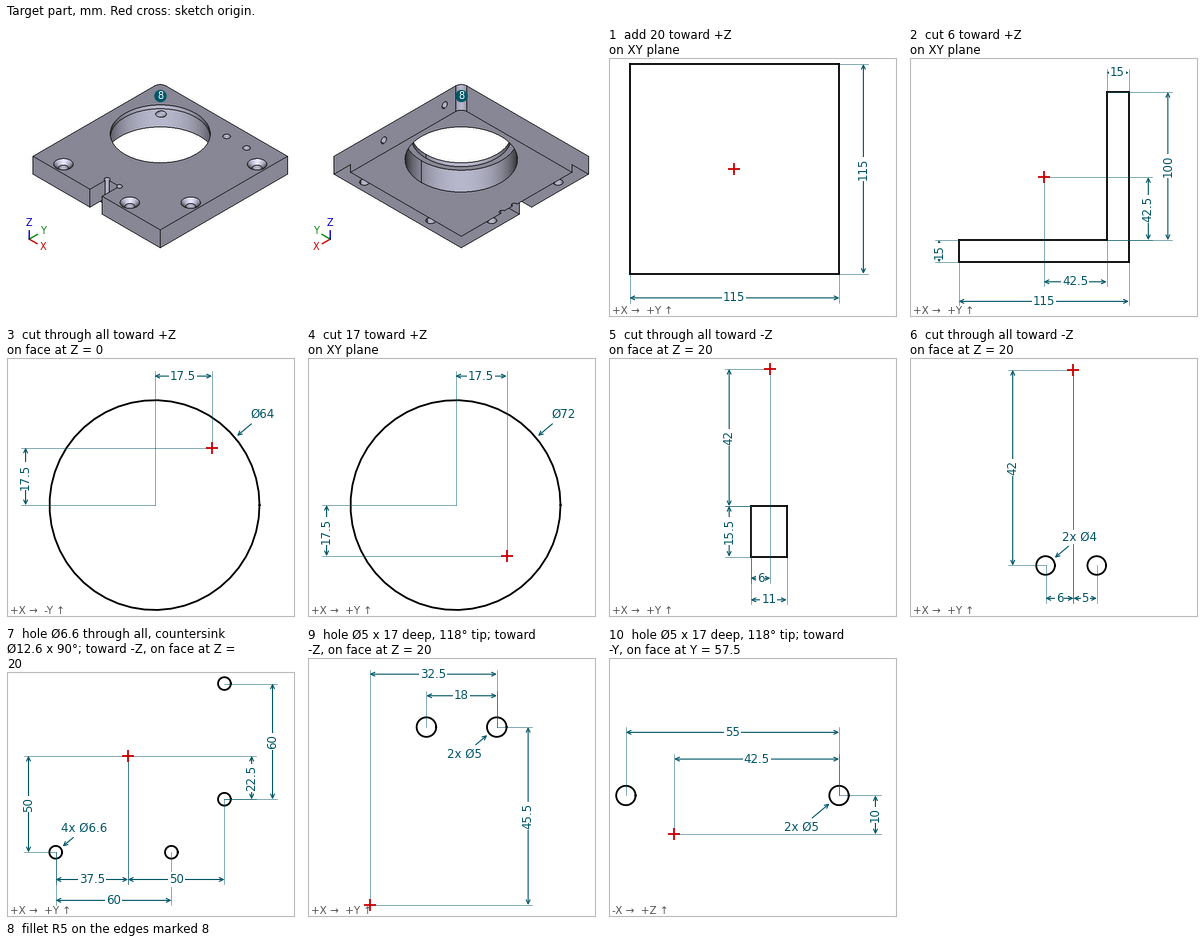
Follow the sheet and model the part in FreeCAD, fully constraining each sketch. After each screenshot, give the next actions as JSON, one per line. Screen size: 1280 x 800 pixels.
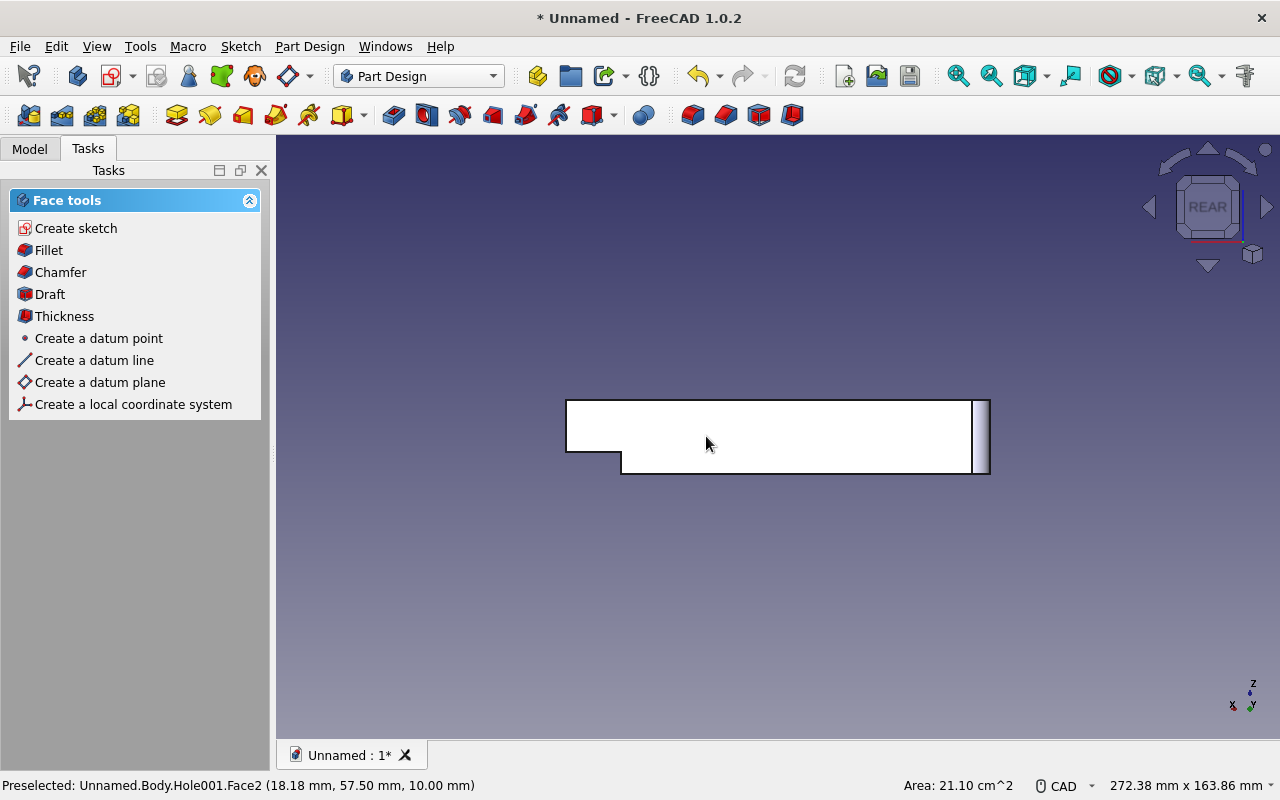
{"action": "left_click", "coordinate": [110, 76]}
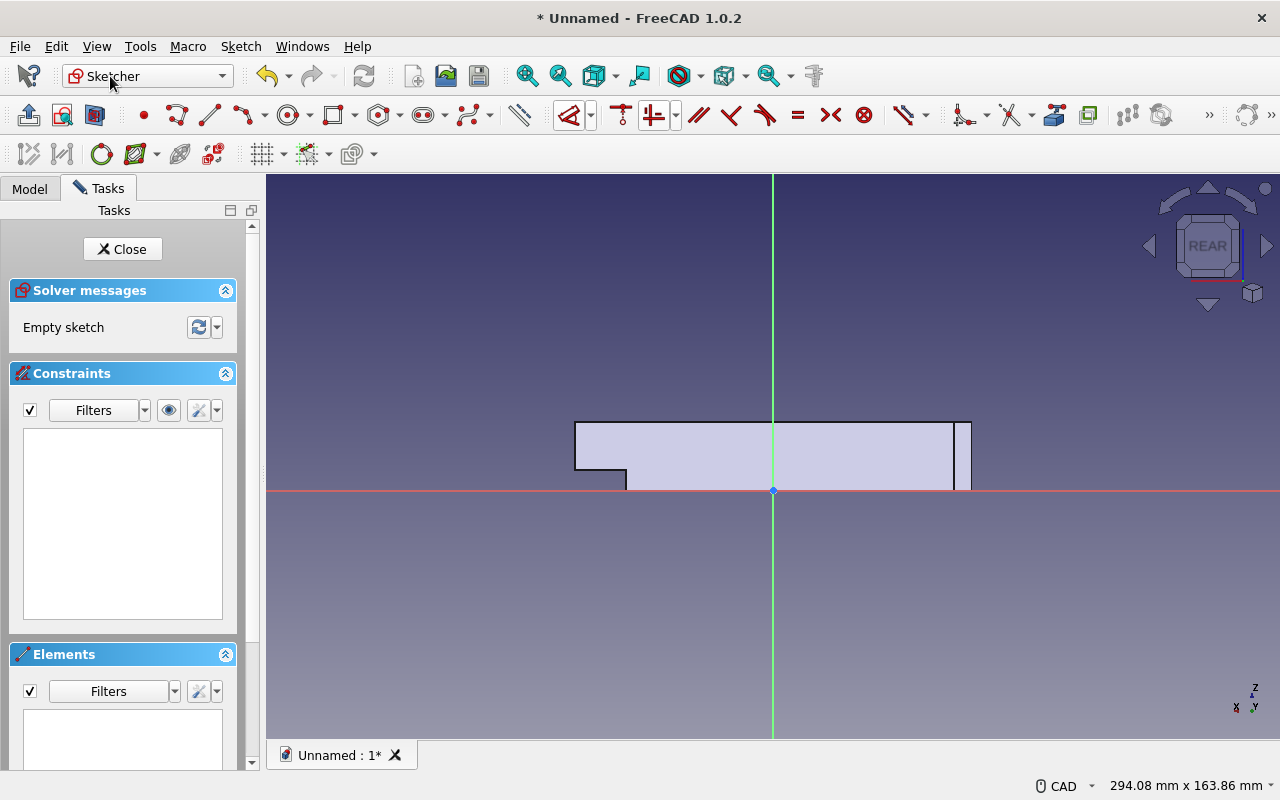
{"action": "scroll", "coordinate": [895, 477], "scroll_direction": "up", "scroll_amount": 5}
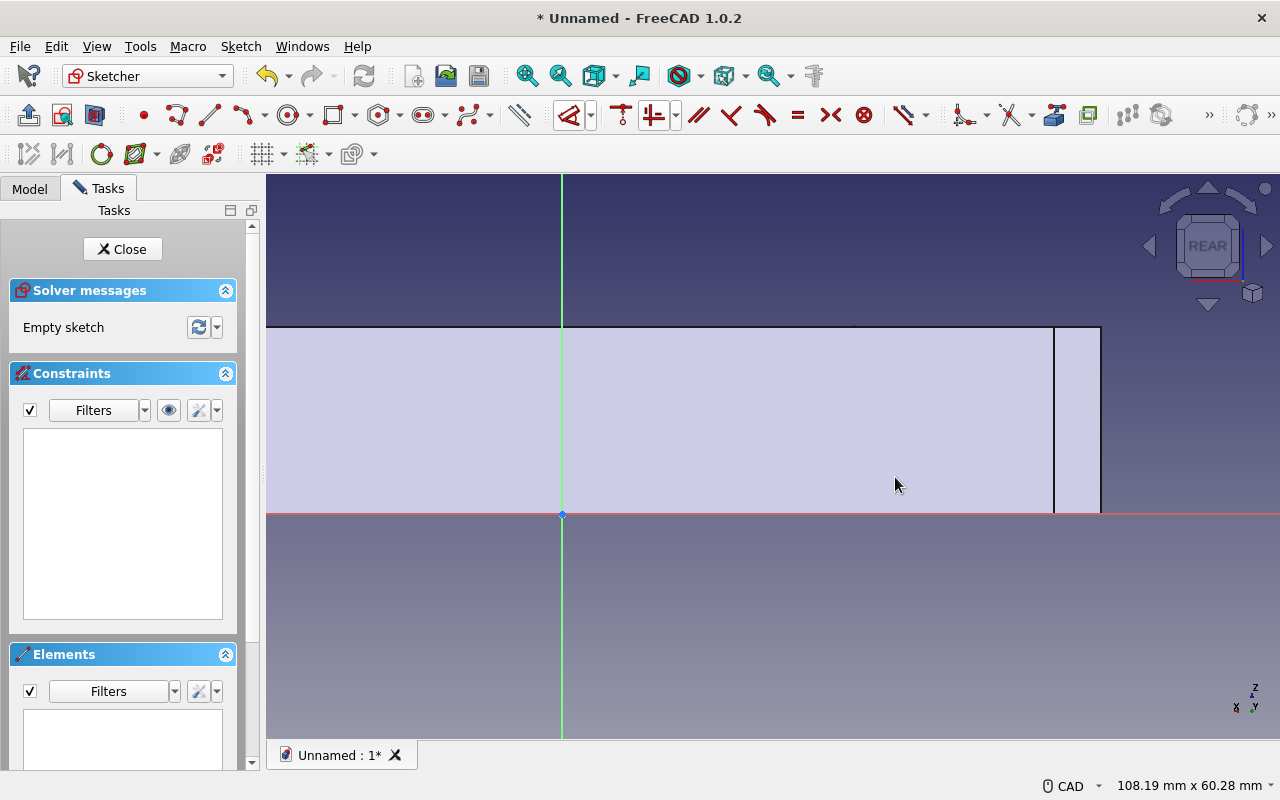
{"action": "key", "text": "g c"}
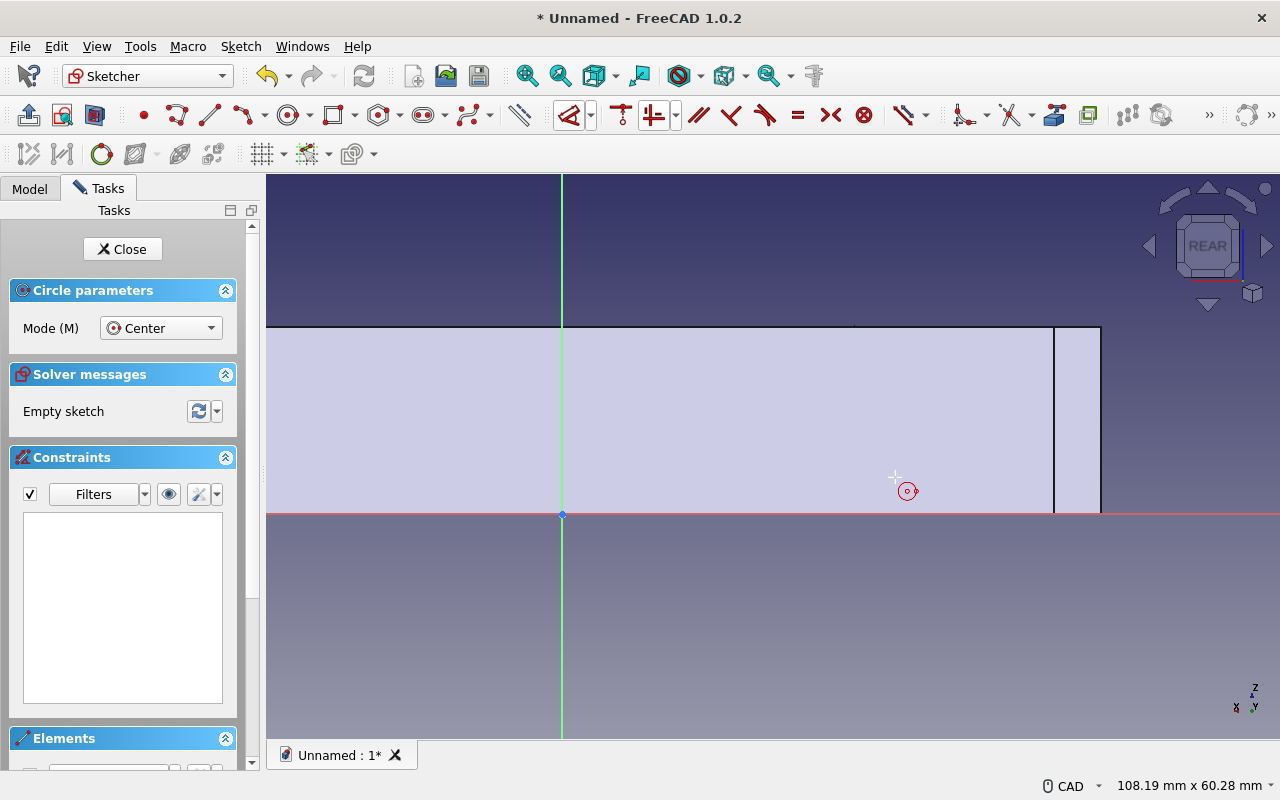
{"action": "left_click", "coordinate": [961, 420]}
{"action": "left_click", "coordinate": [977, 404]}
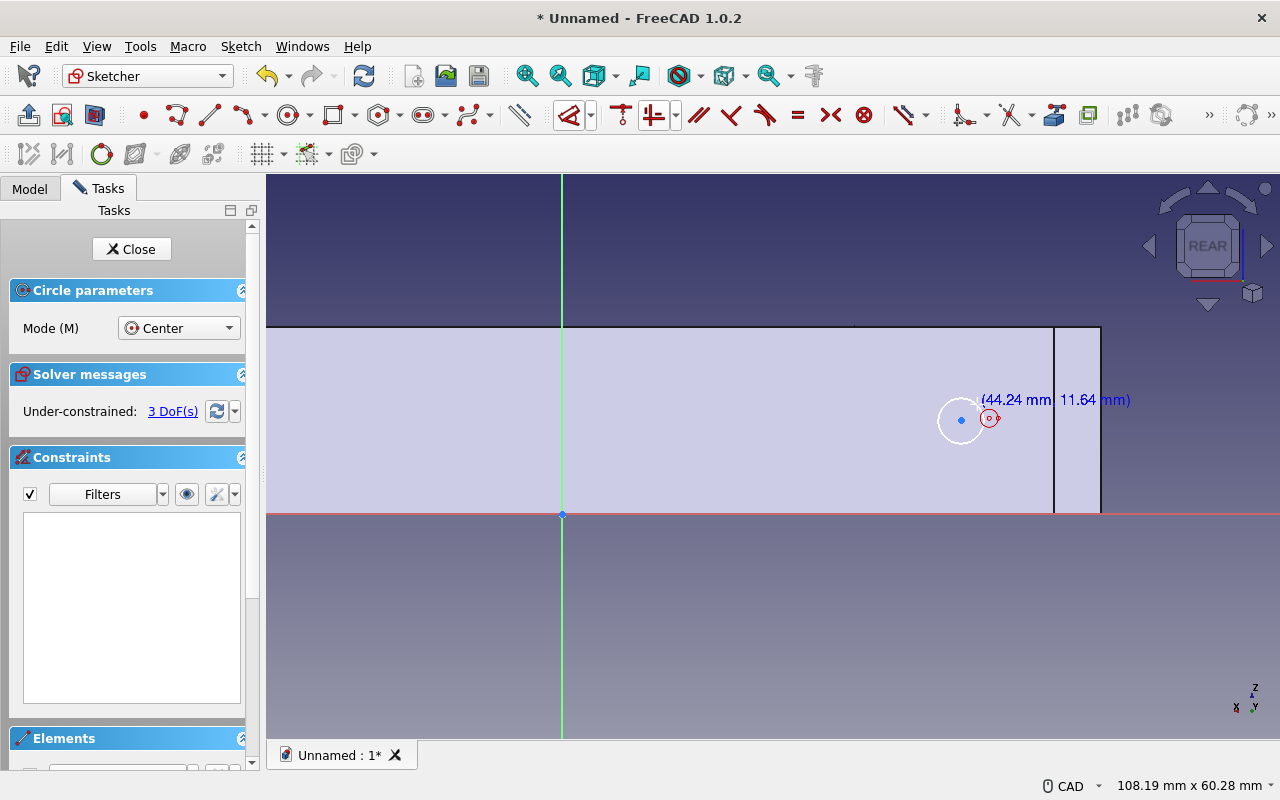
{"action": "left_click", "coordinate": [445, 420]}
{"action": "left_click", "coordinate": [462, 404]}
{"action": "key", "text": "Escape"}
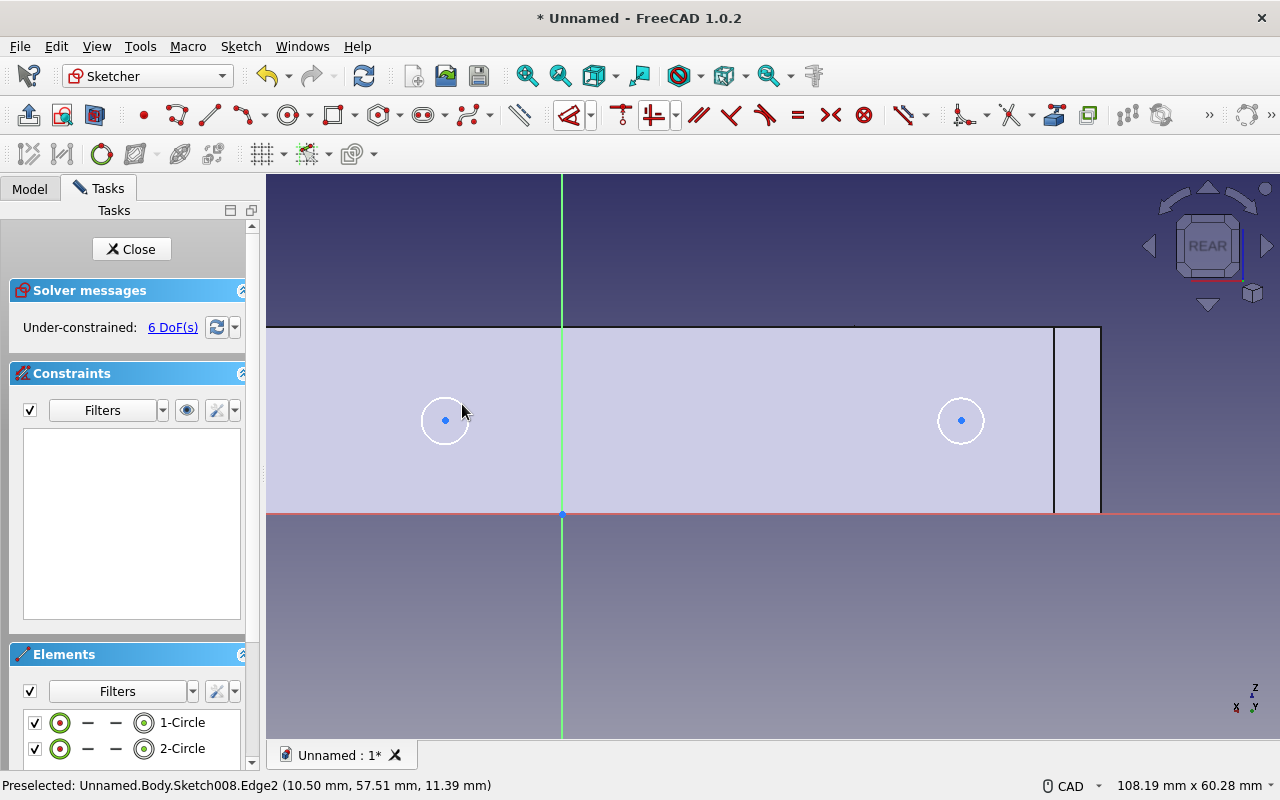
{"action": "left_click", "coordinate": [977, 405]}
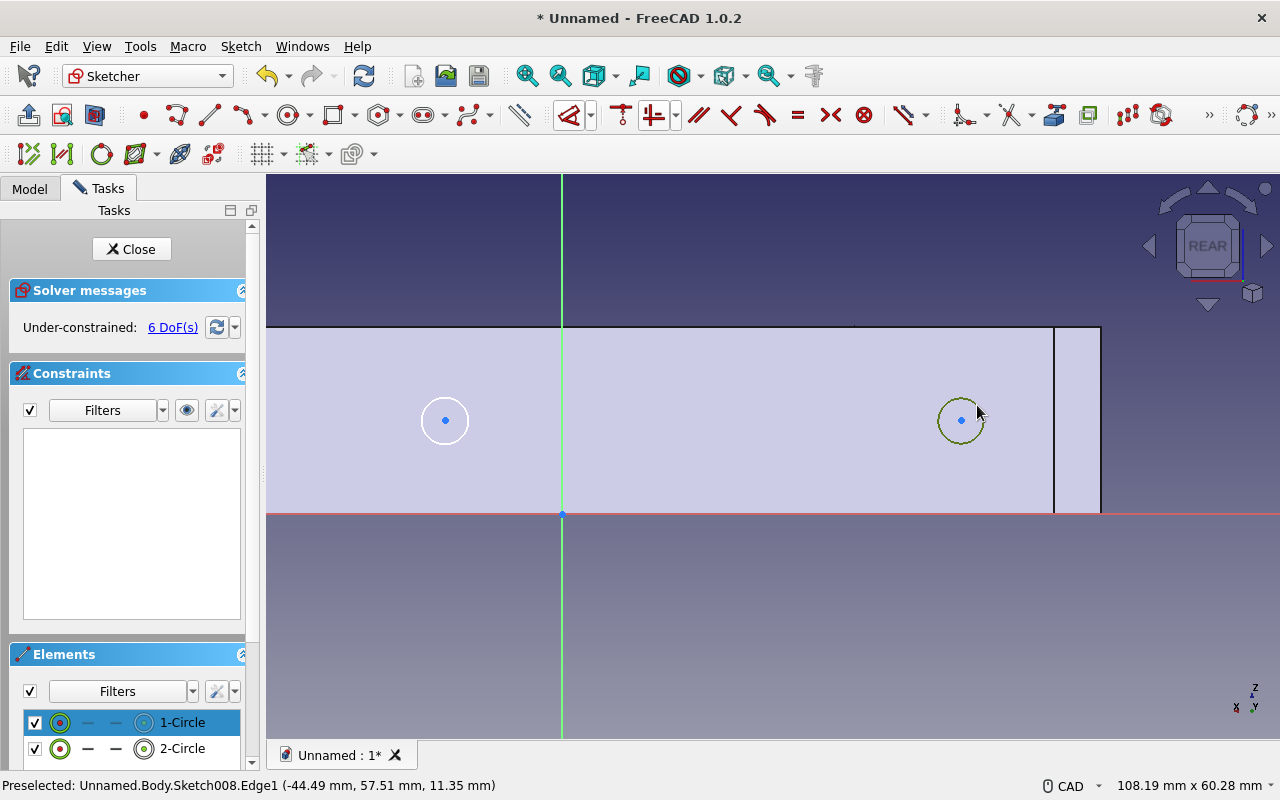
{"action": "left_click", "coordinate": [461, 404]}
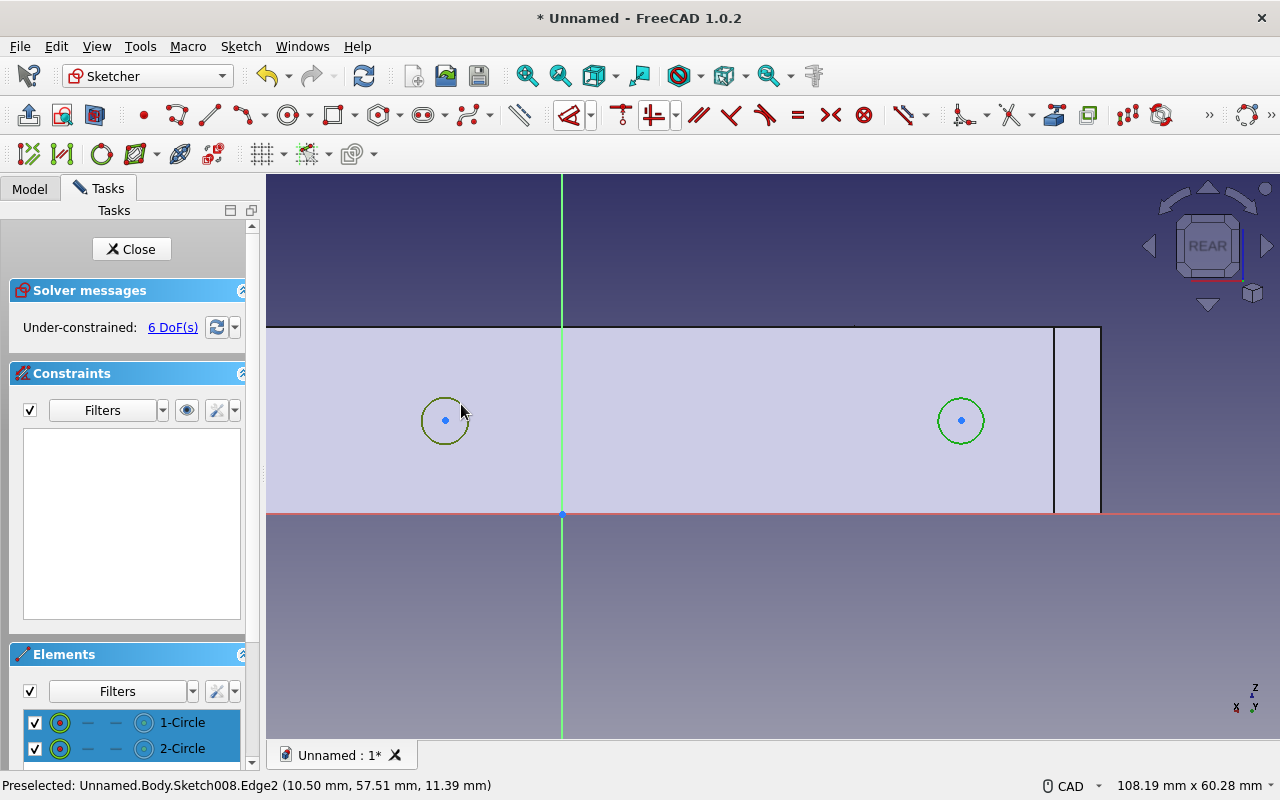
{"action": "key", "text": "e"}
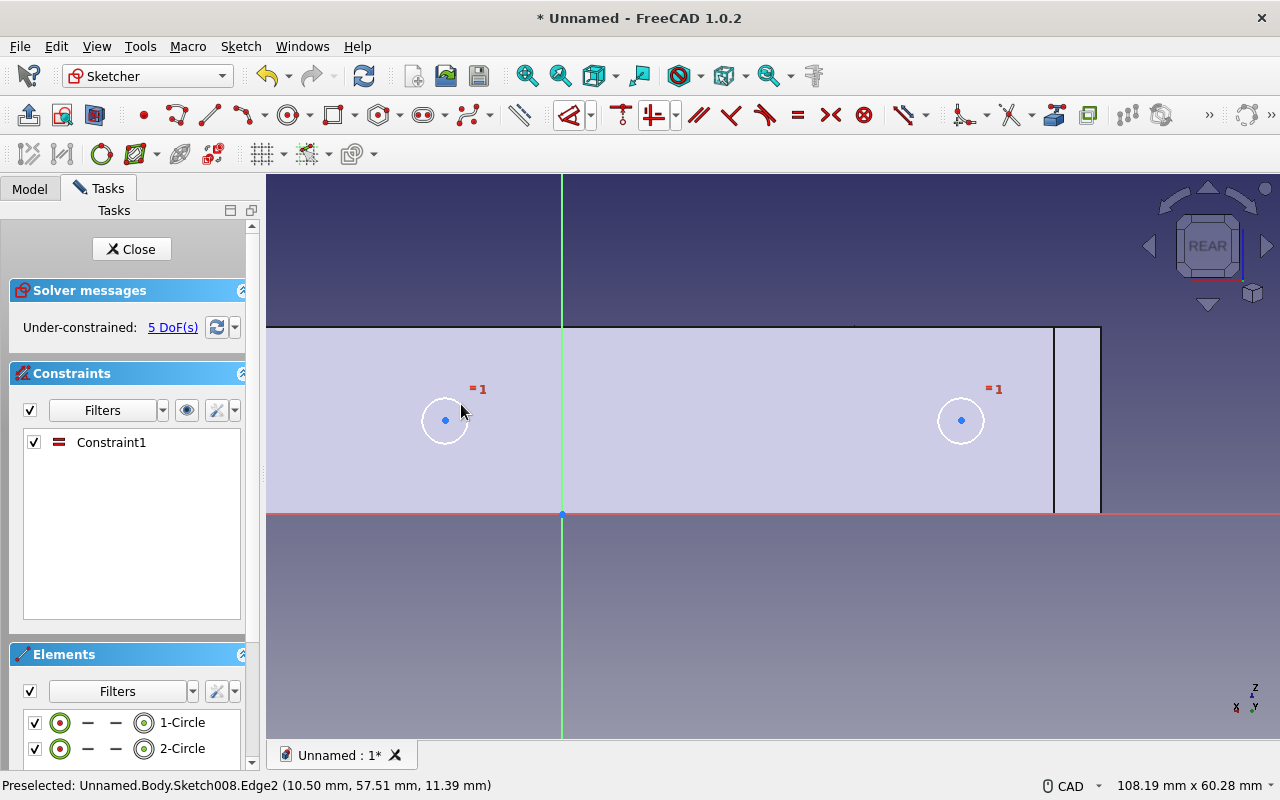
{"action": "left_click", "coordinate": [961, 421]}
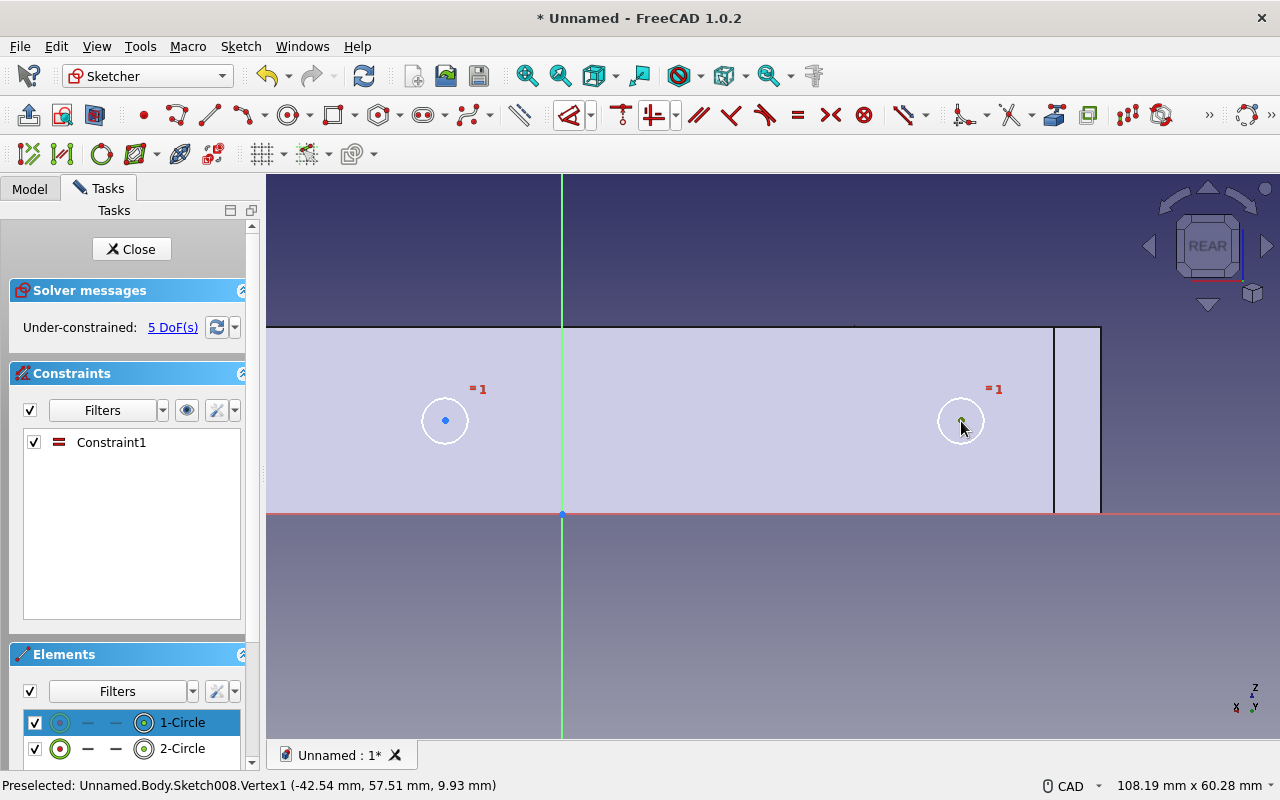
{"action": "left_click", "coordinate": [445, 421]}